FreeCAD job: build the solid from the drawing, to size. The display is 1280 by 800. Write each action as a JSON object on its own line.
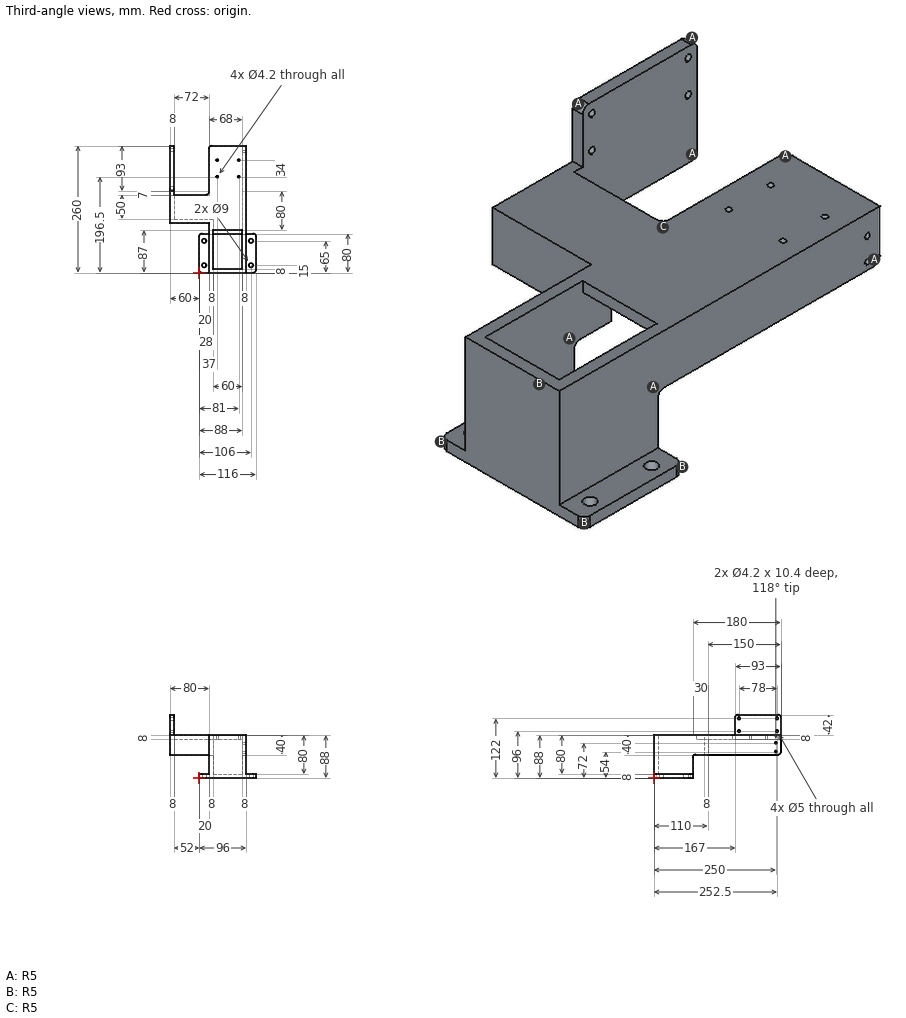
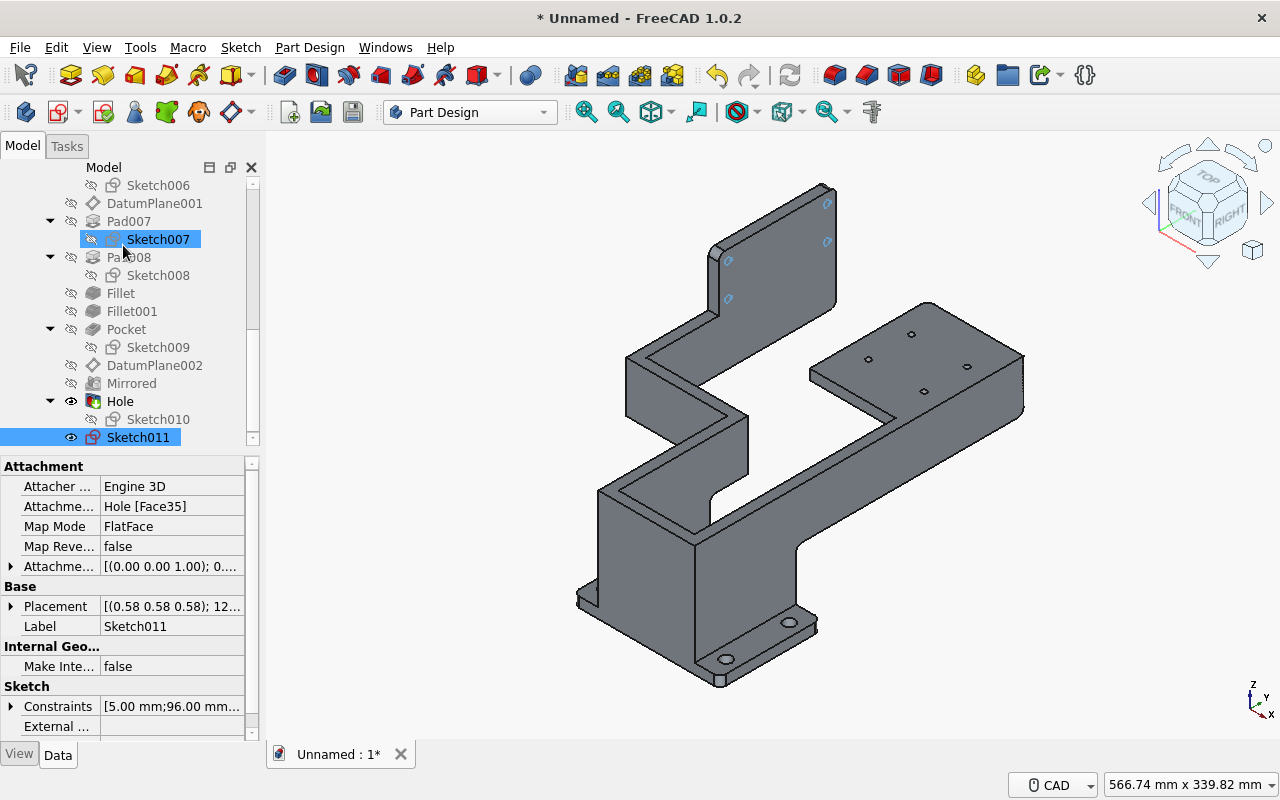
{"action": "left_click", "coordinate": [318, 76]}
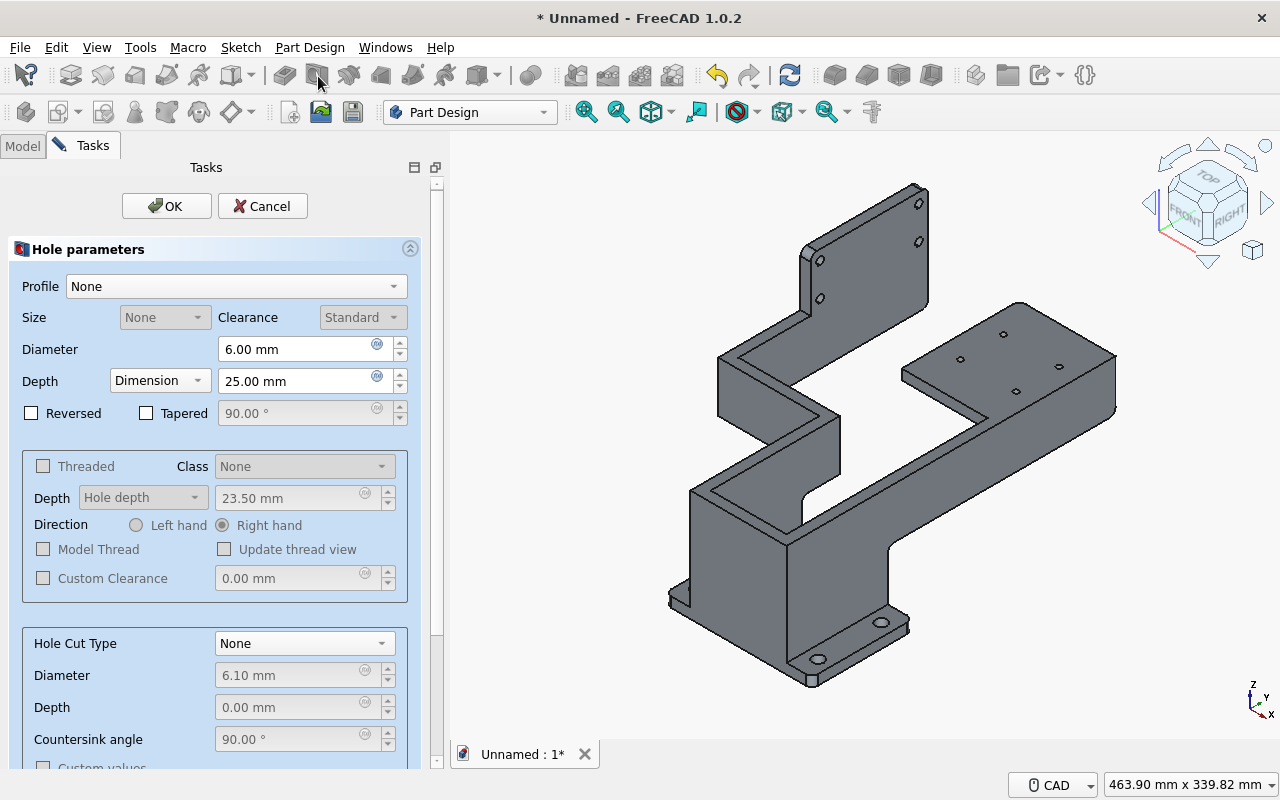
{"action": "triple_click", "coordinate": [305, 349]}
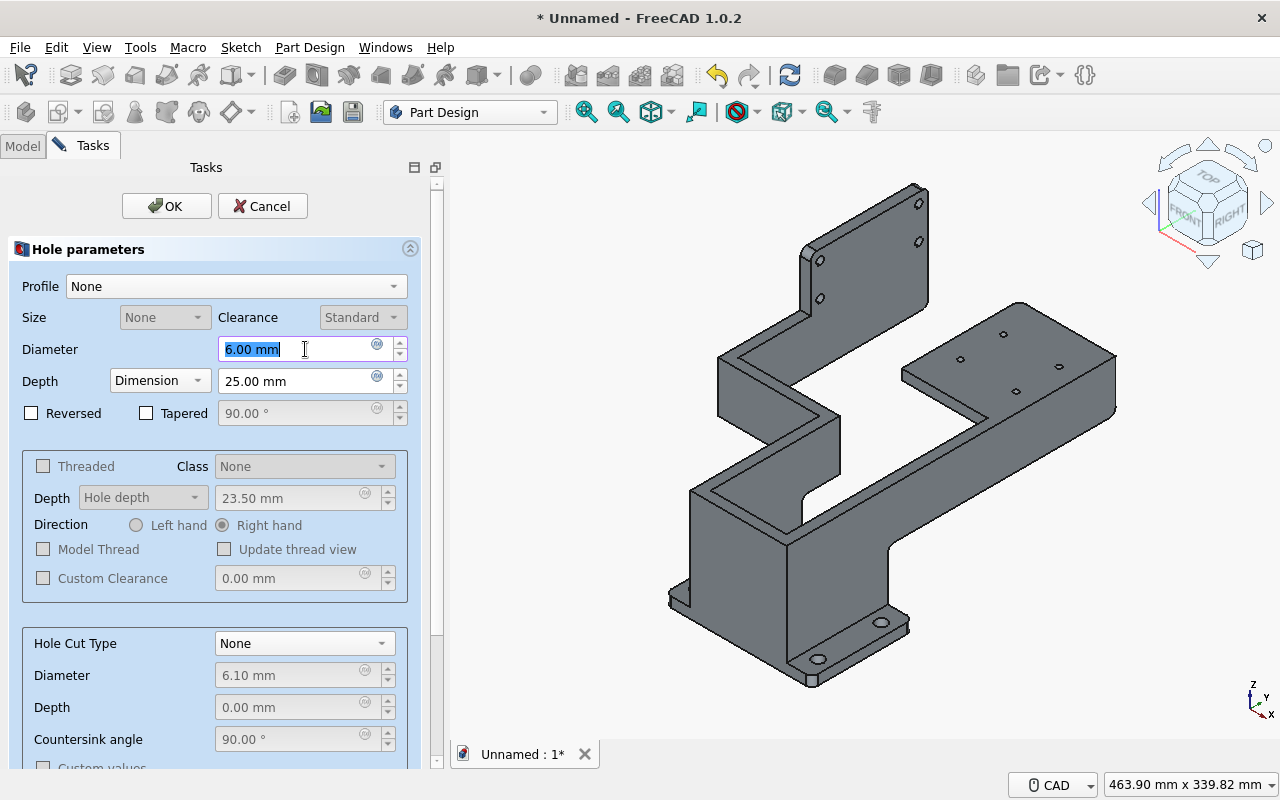
{"action": "type", "text": "5"}
{"action": "key", "text": "Tab"}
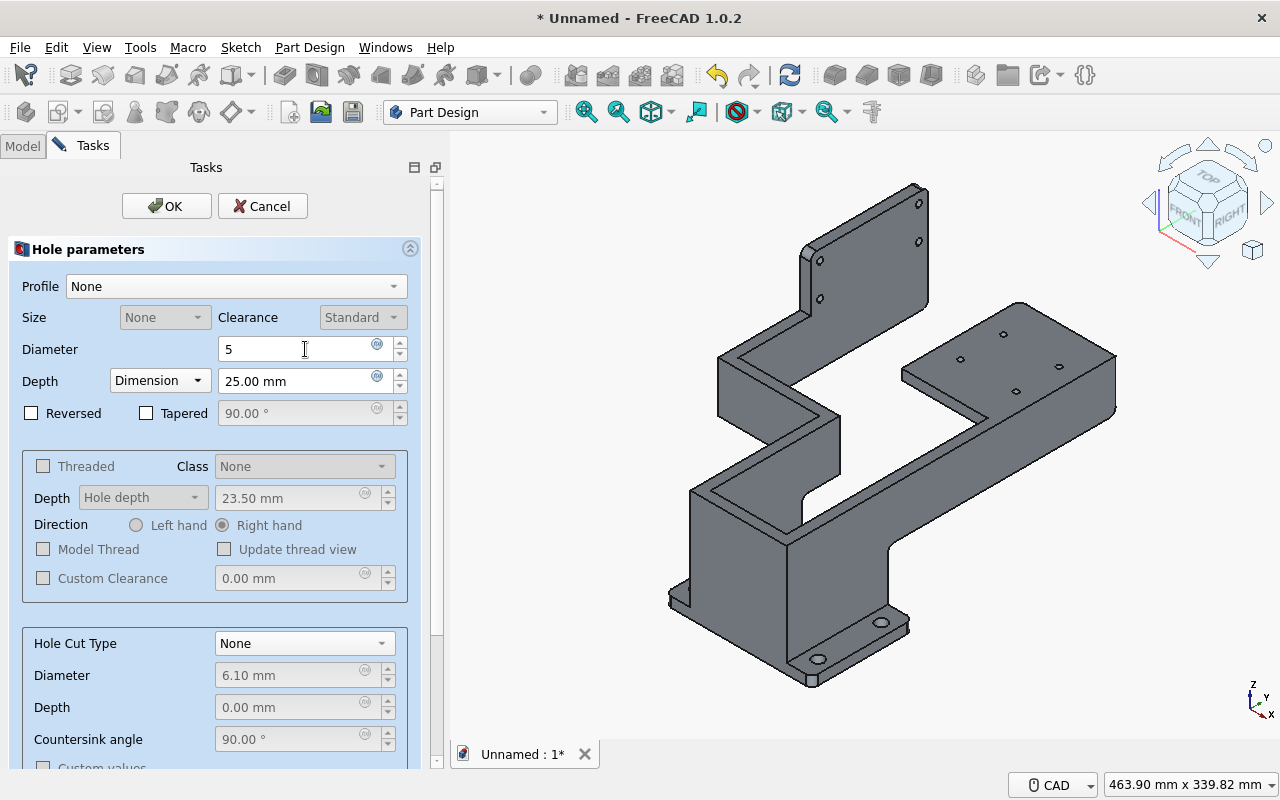
{"action": "left_click", "coordinate": [161, 380]}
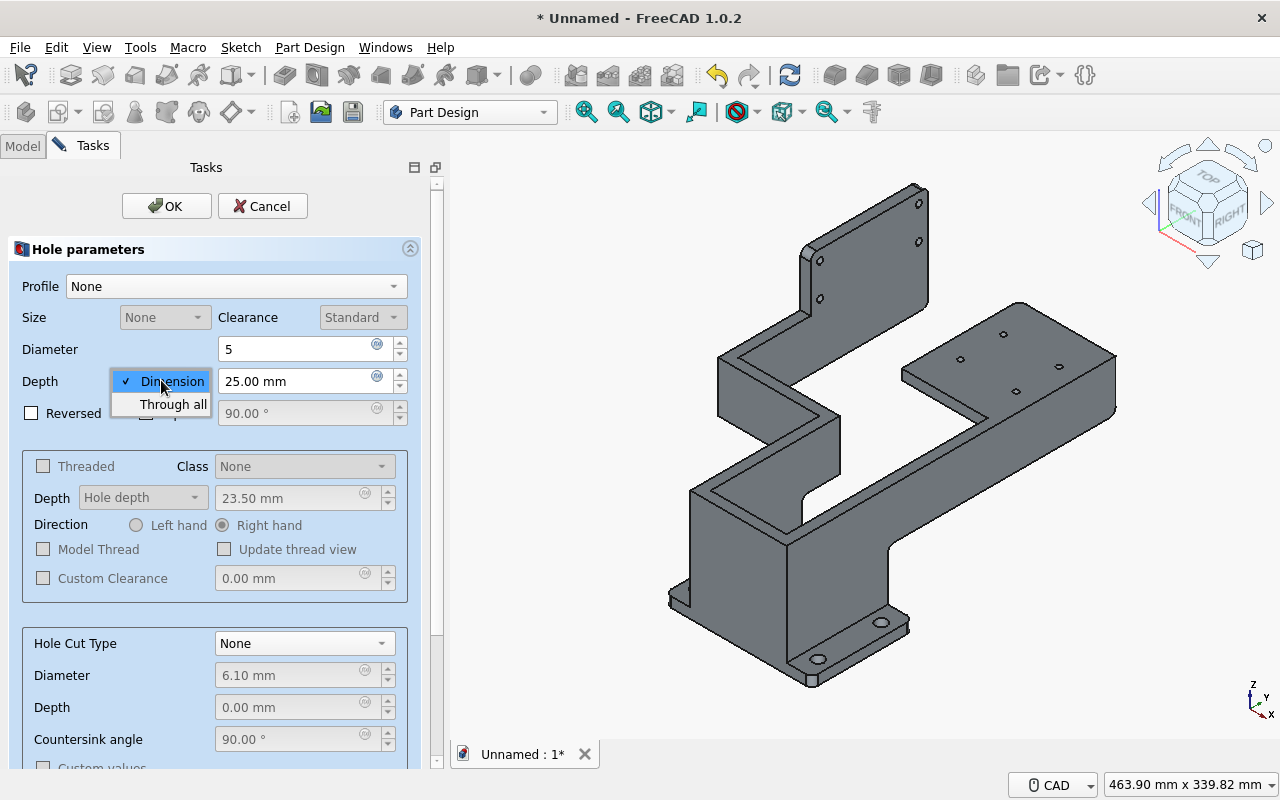
{"action": "left_click", "coordinate": [160, 404]}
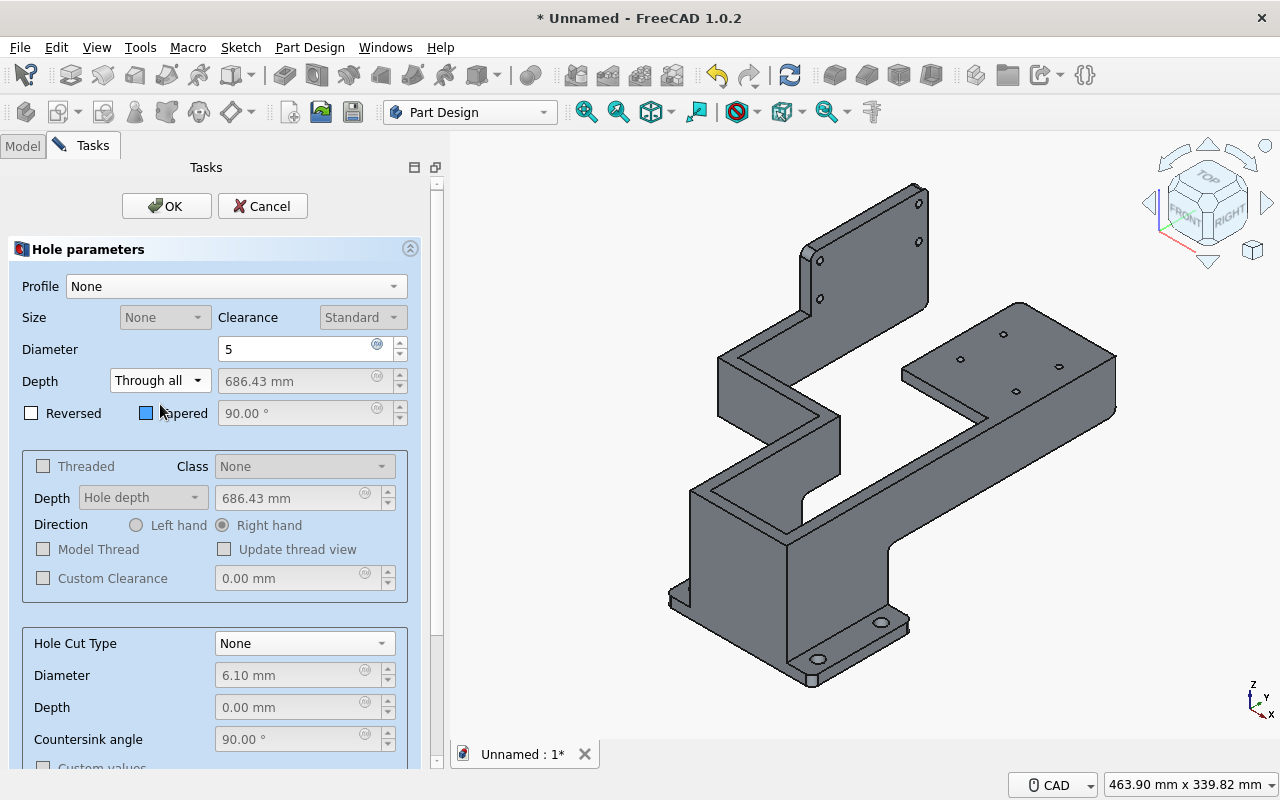
{"action": "left_click", "coordinate": [167, 206]}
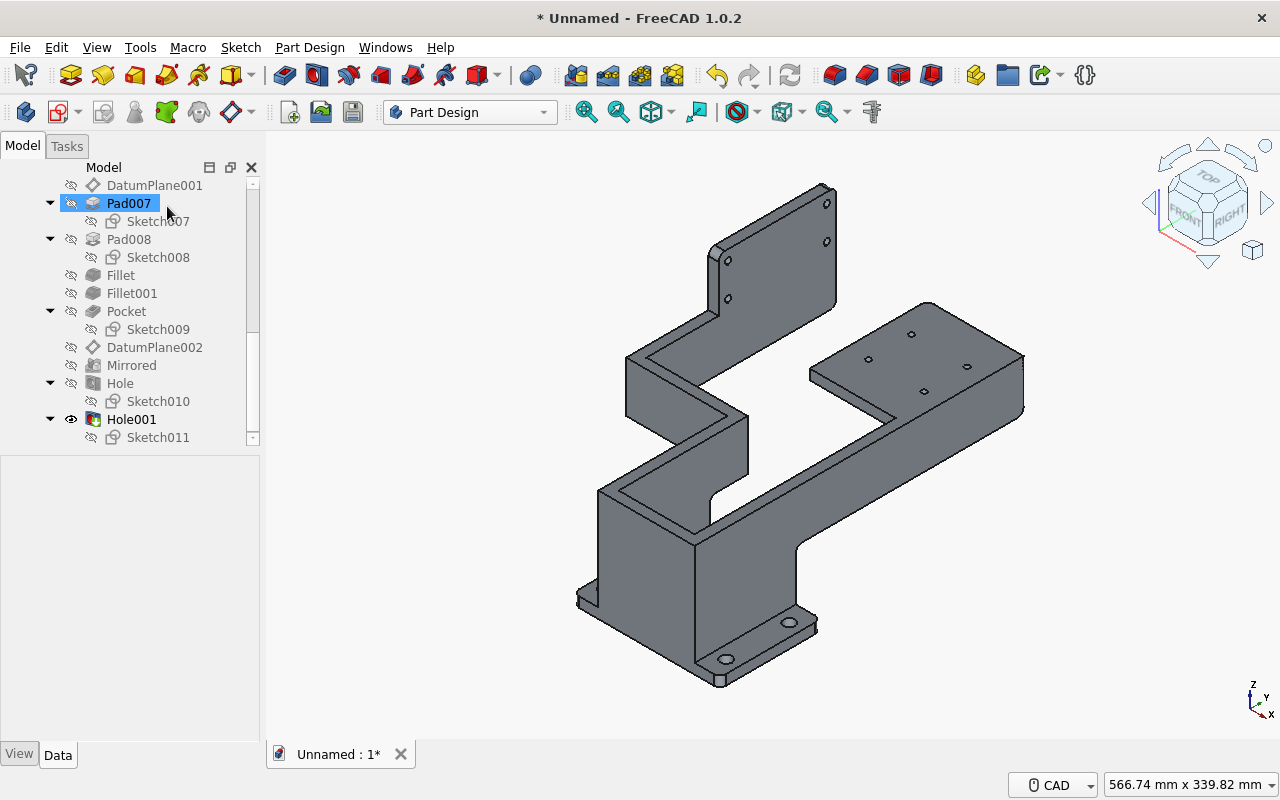
{"action": "left_click", "coordinate": [765, 546]}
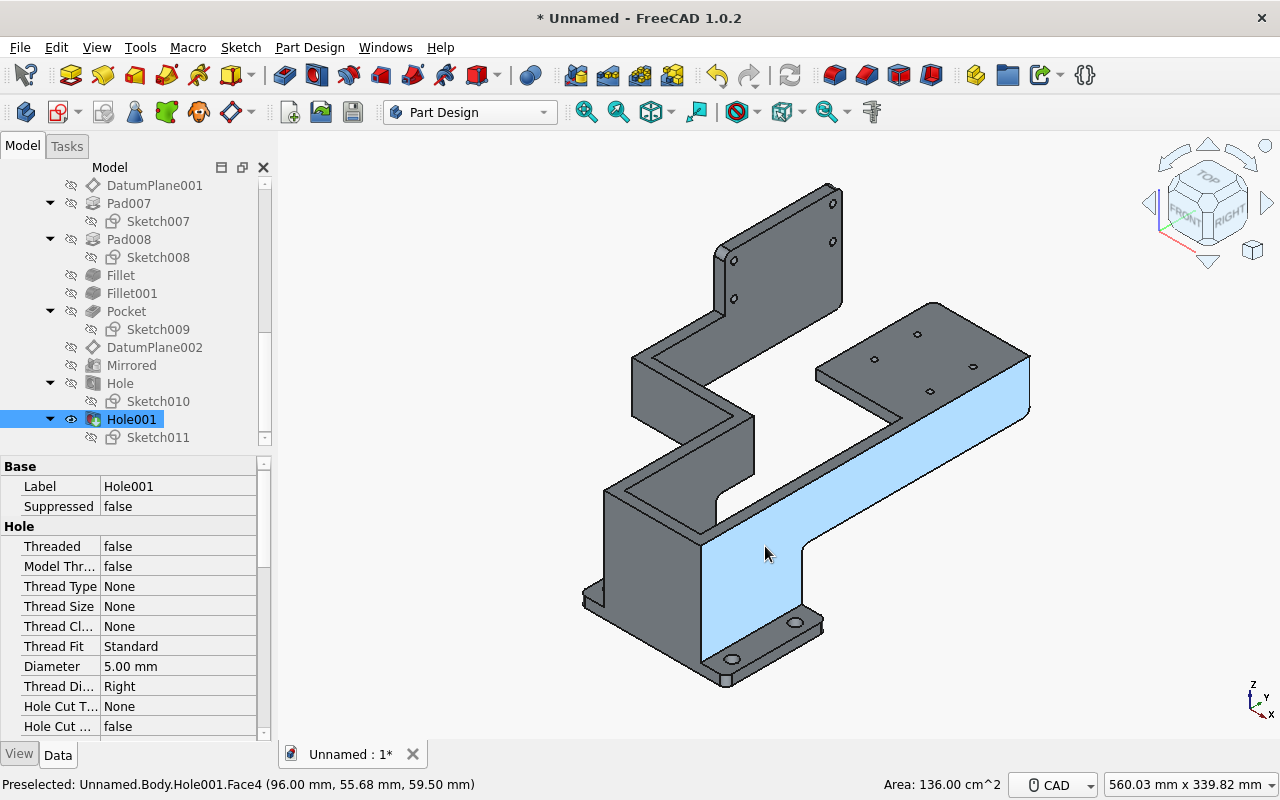
{"action": "left_click", "coordinate": [58, 112]}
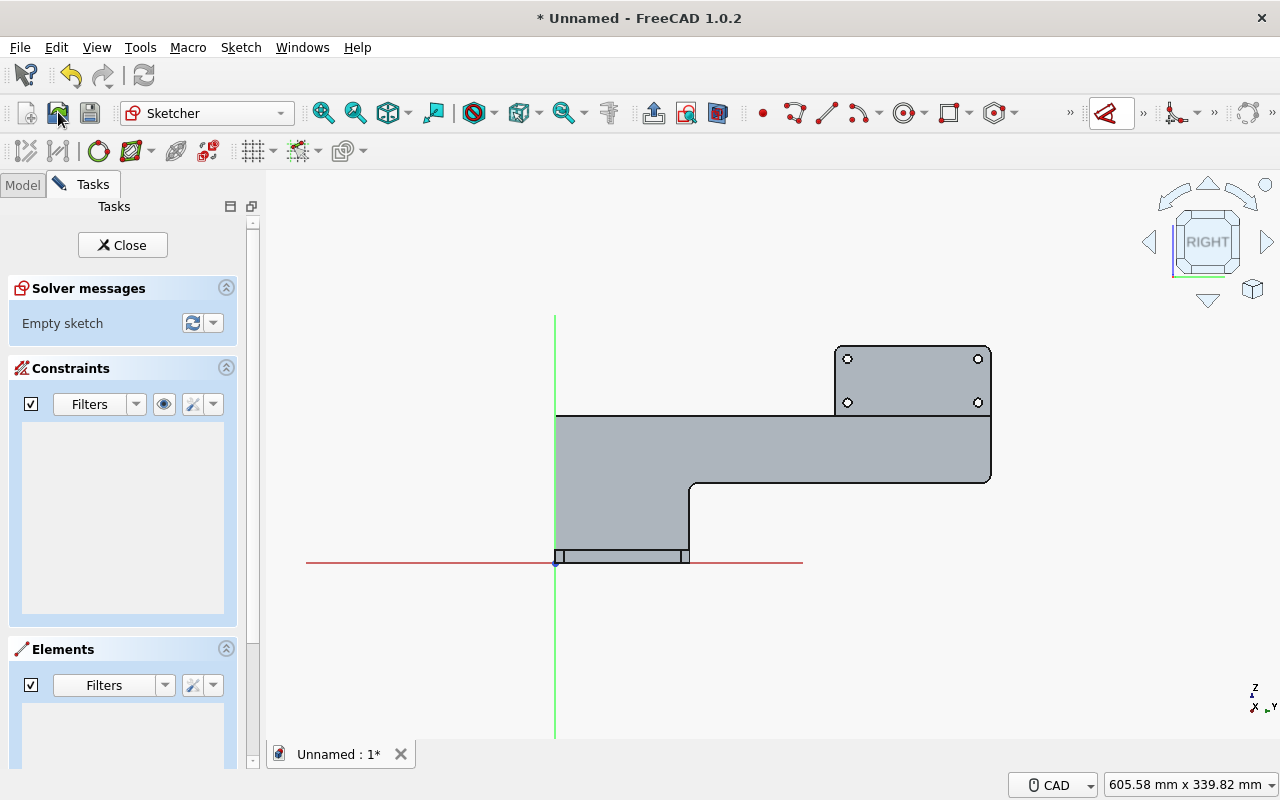
{"action": "scroll", "coordinate": [1008, 458], "scroll_direction": "up", "scroll_amount": 11}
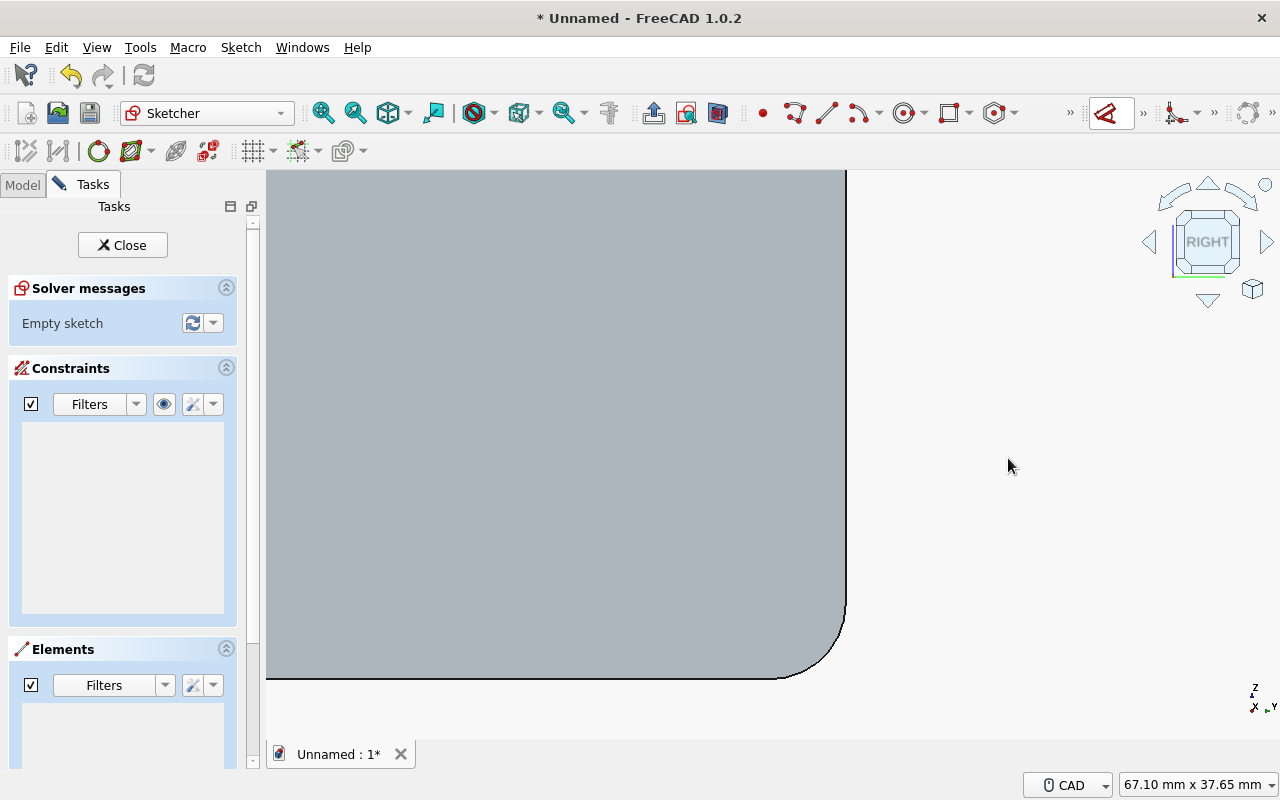
{"action": "left_click", "coordinate": [904, 114]}